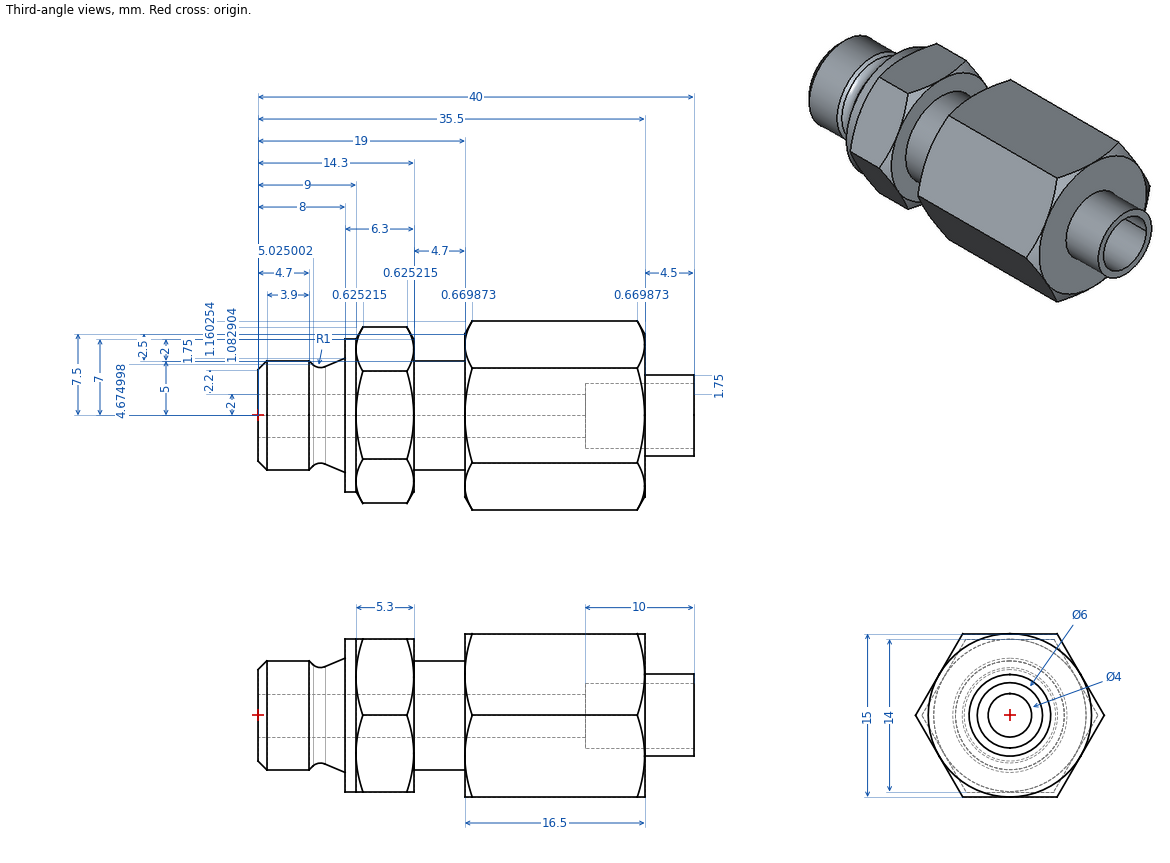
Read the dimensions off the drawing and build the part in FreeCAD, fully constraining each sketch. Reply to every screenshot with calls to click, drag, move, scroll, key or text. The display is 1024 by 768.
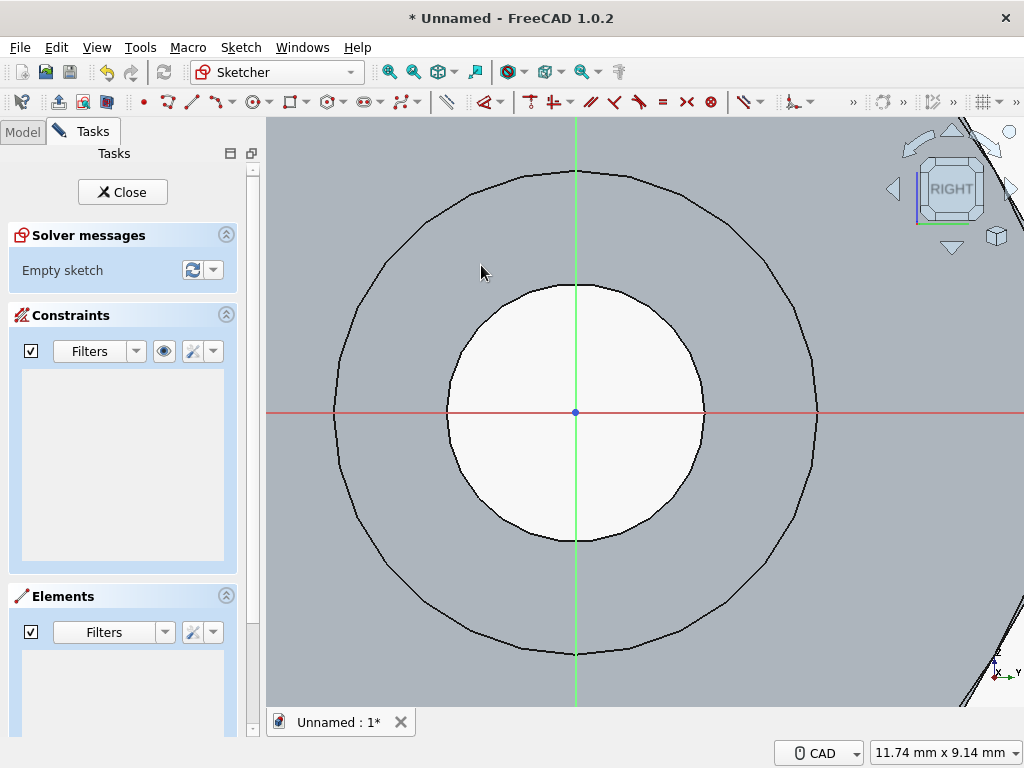
click(254, 102)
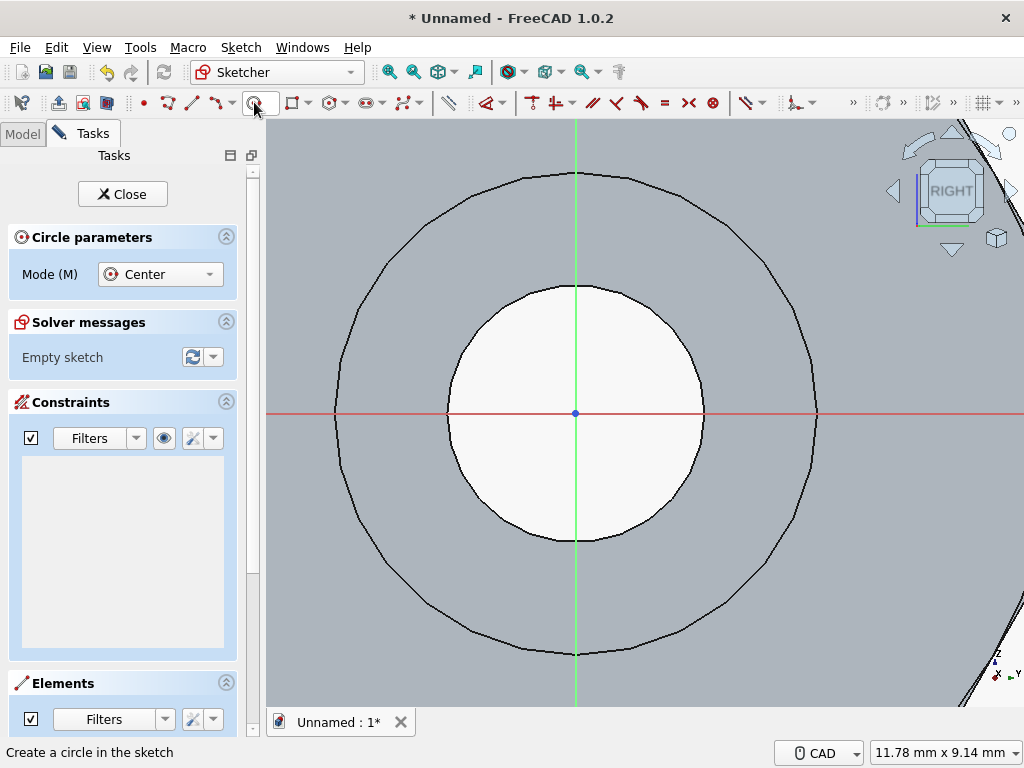
click(576, 414)
click(712, 277)
key(Escape)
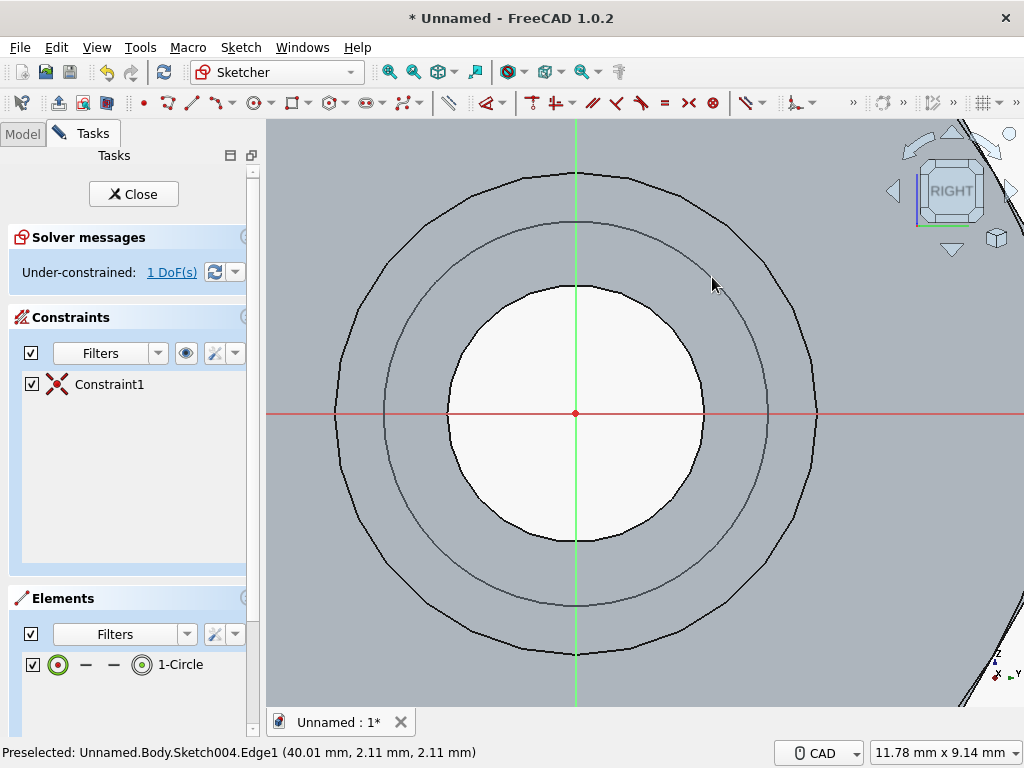
click(486, 104)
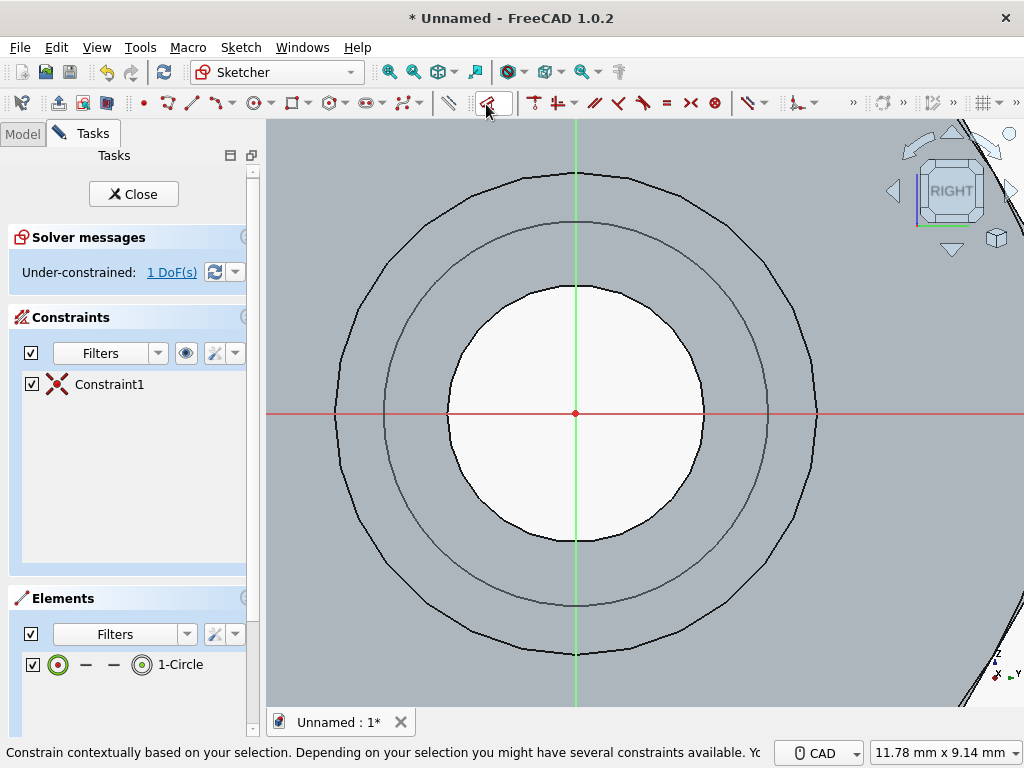
click(711, 277)
click(733, 254)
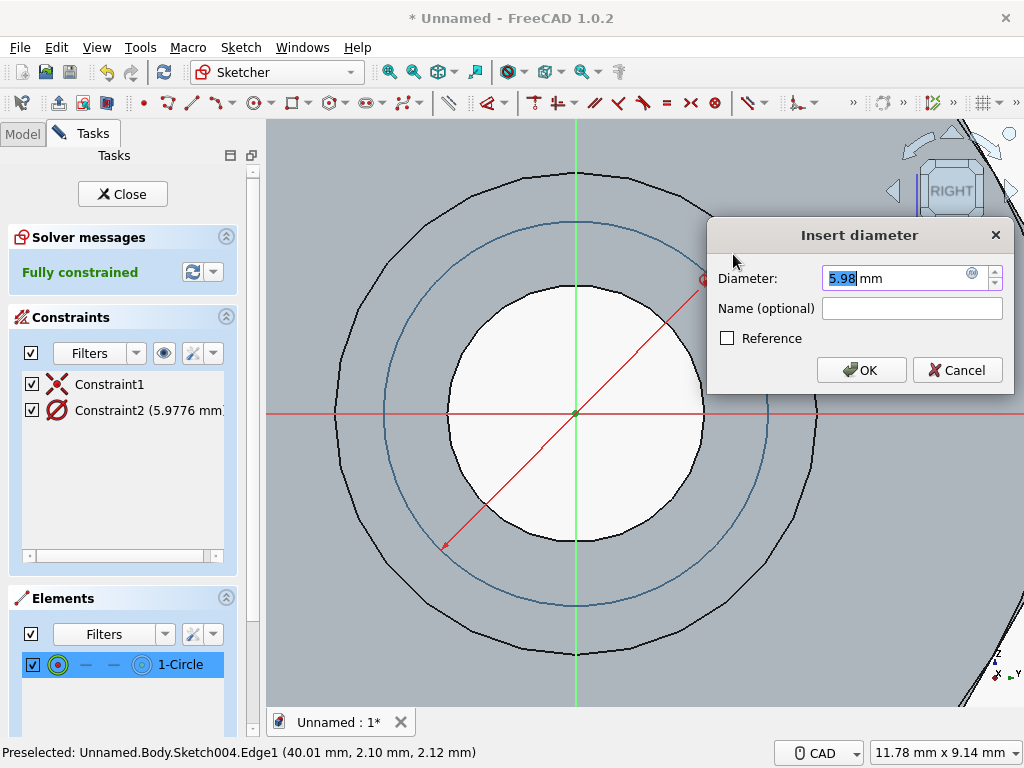
text(6)
key(Return)
key(Escape)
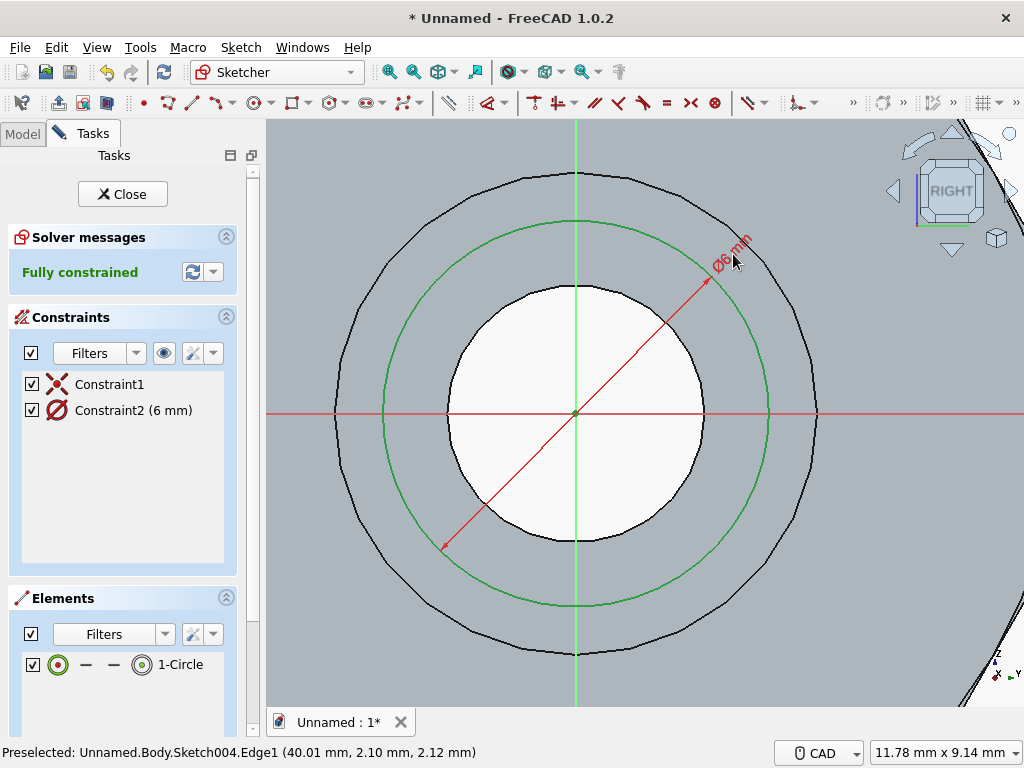
click(123, 194)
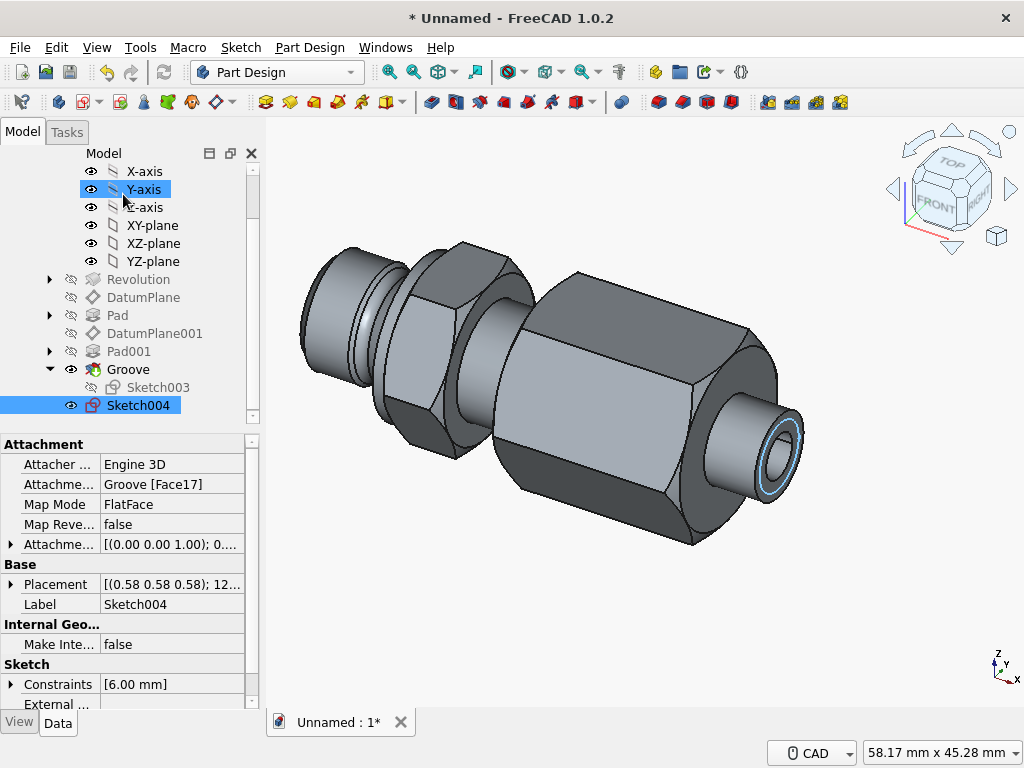
click(432, 102)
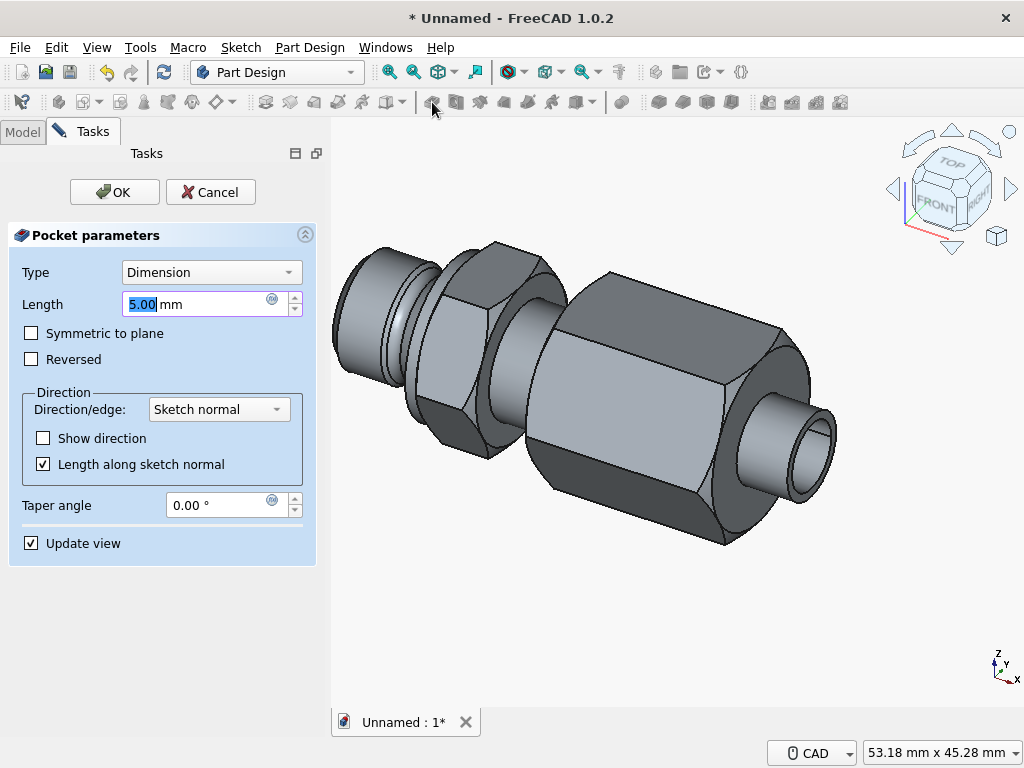
text(10)
key(Tab)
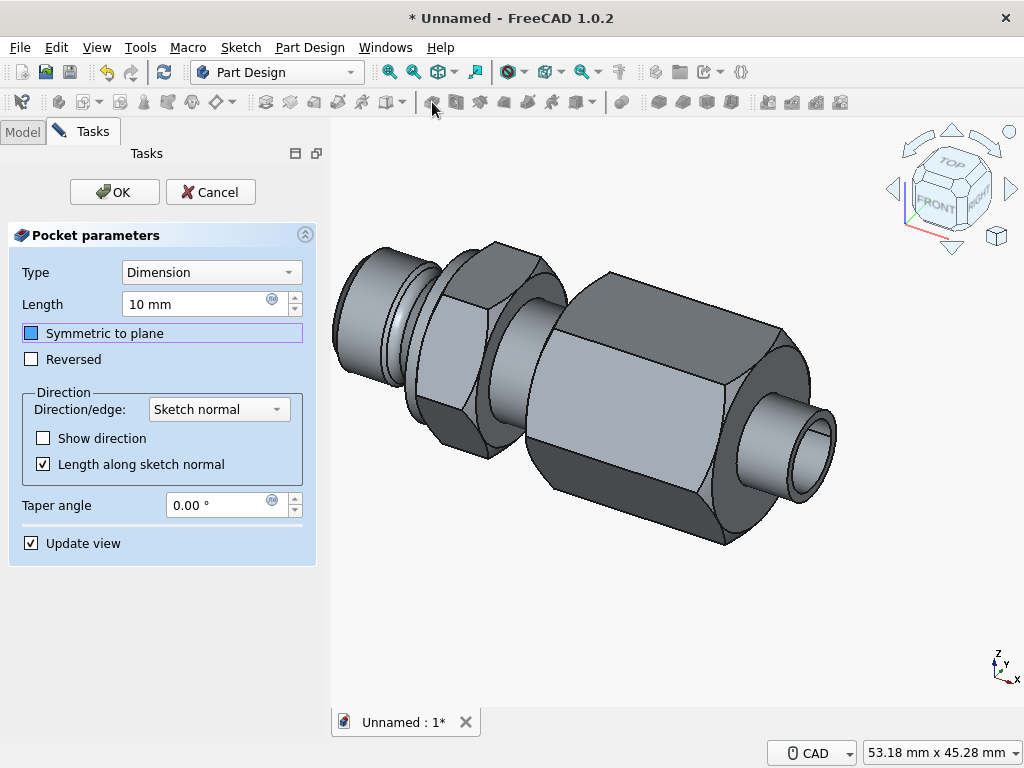
click(115, 192)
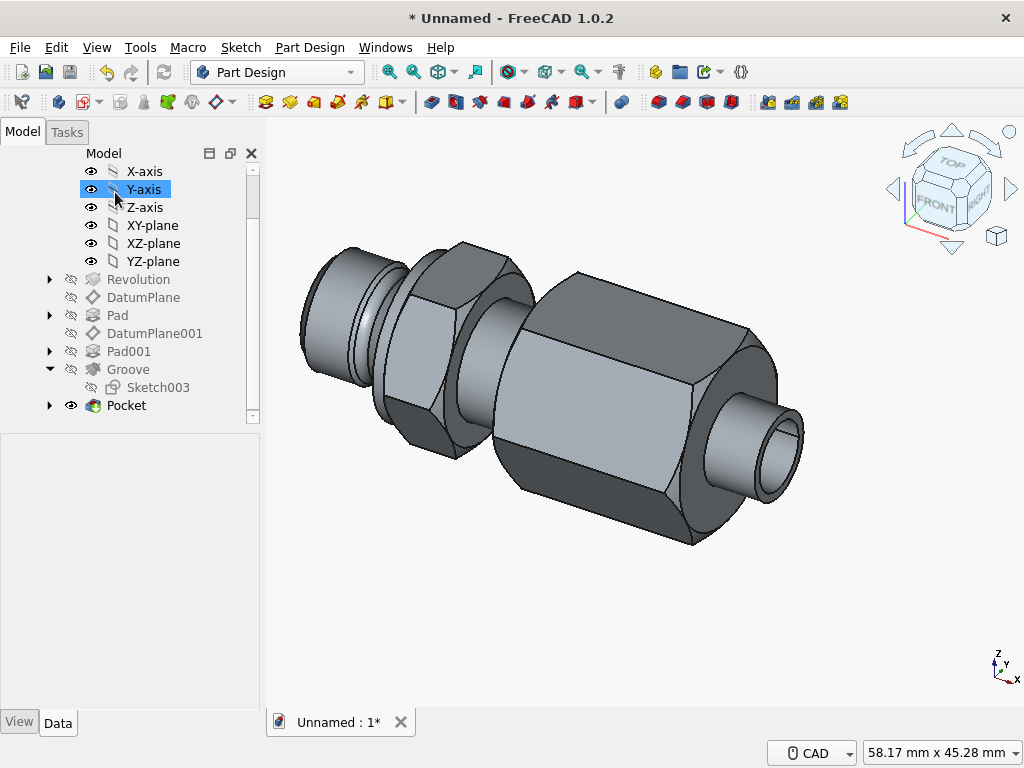
key(0)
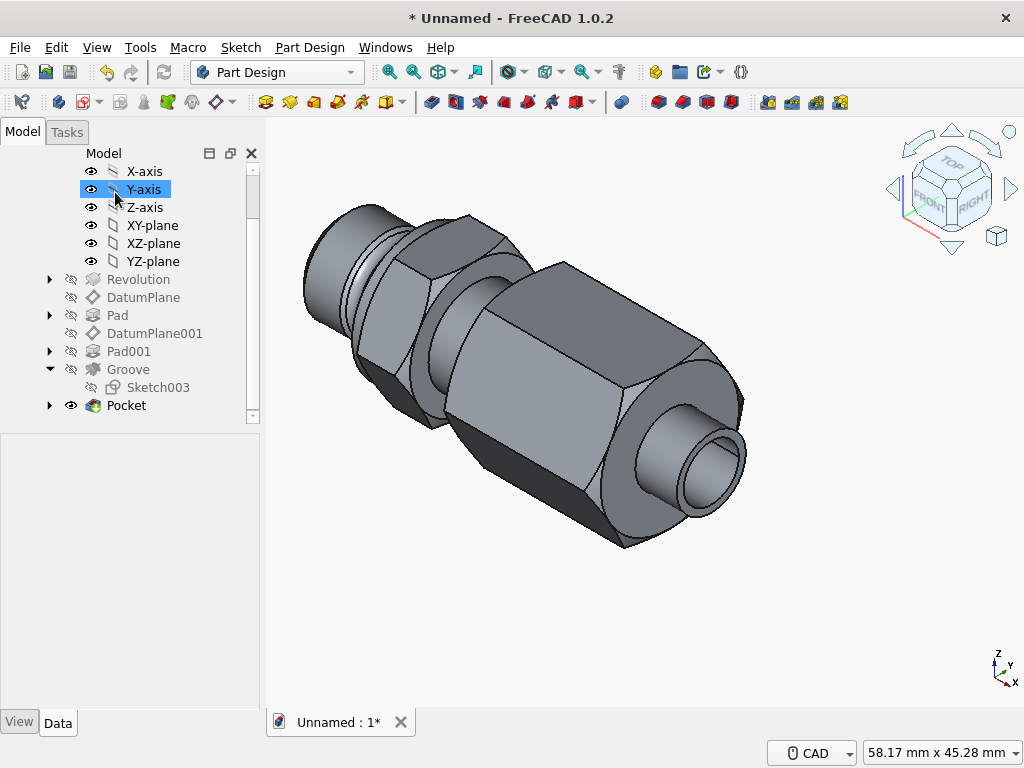
key(v)
key(f)